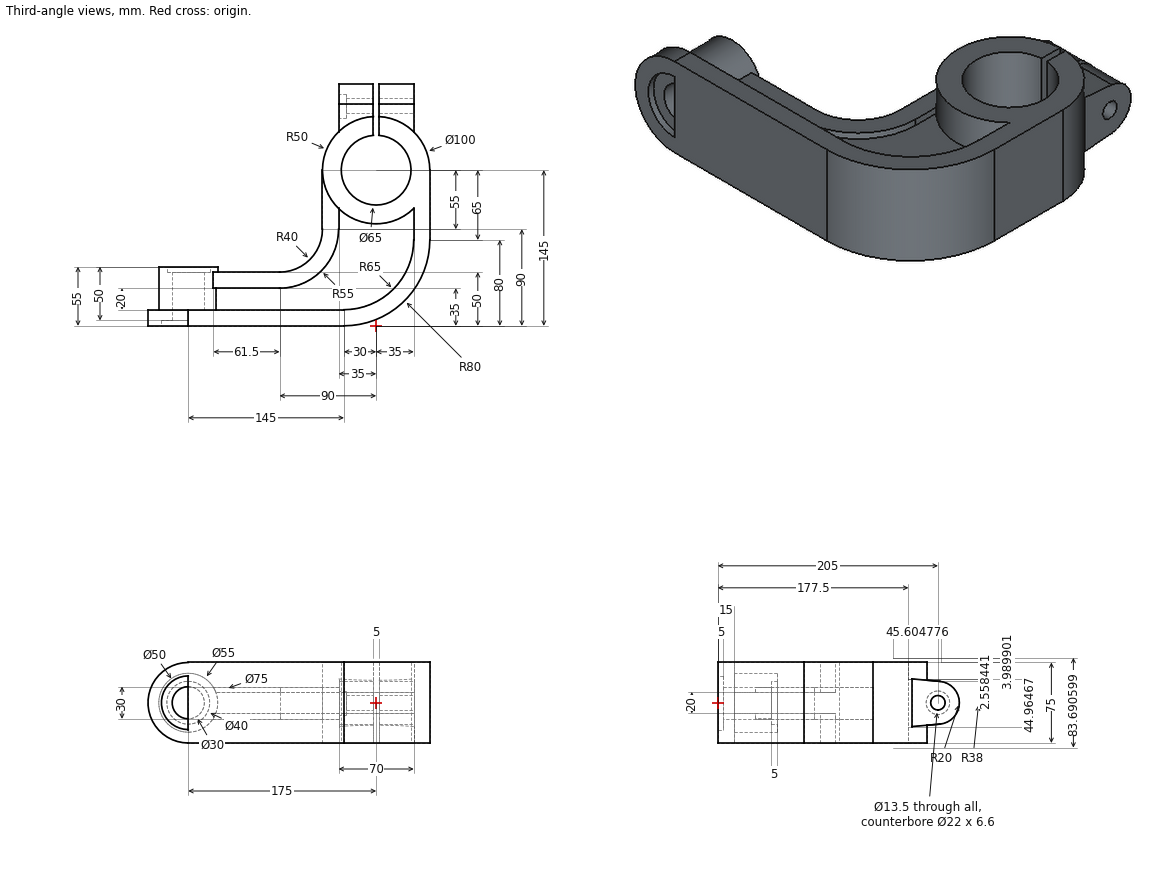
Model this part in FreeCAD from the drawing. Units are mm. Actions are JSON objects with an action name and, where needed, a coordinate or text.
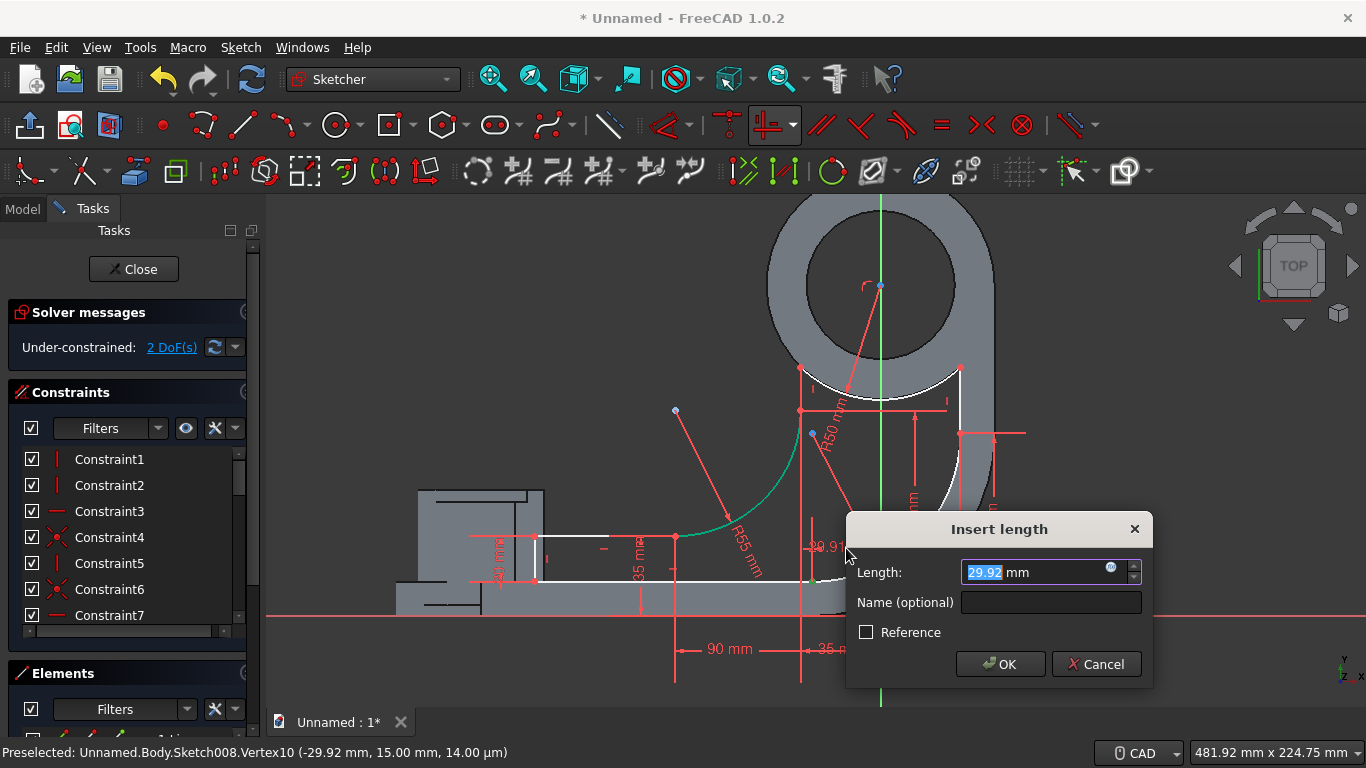
{"action": "type", "text": "30"}
{"action": "key", "text": "Return"}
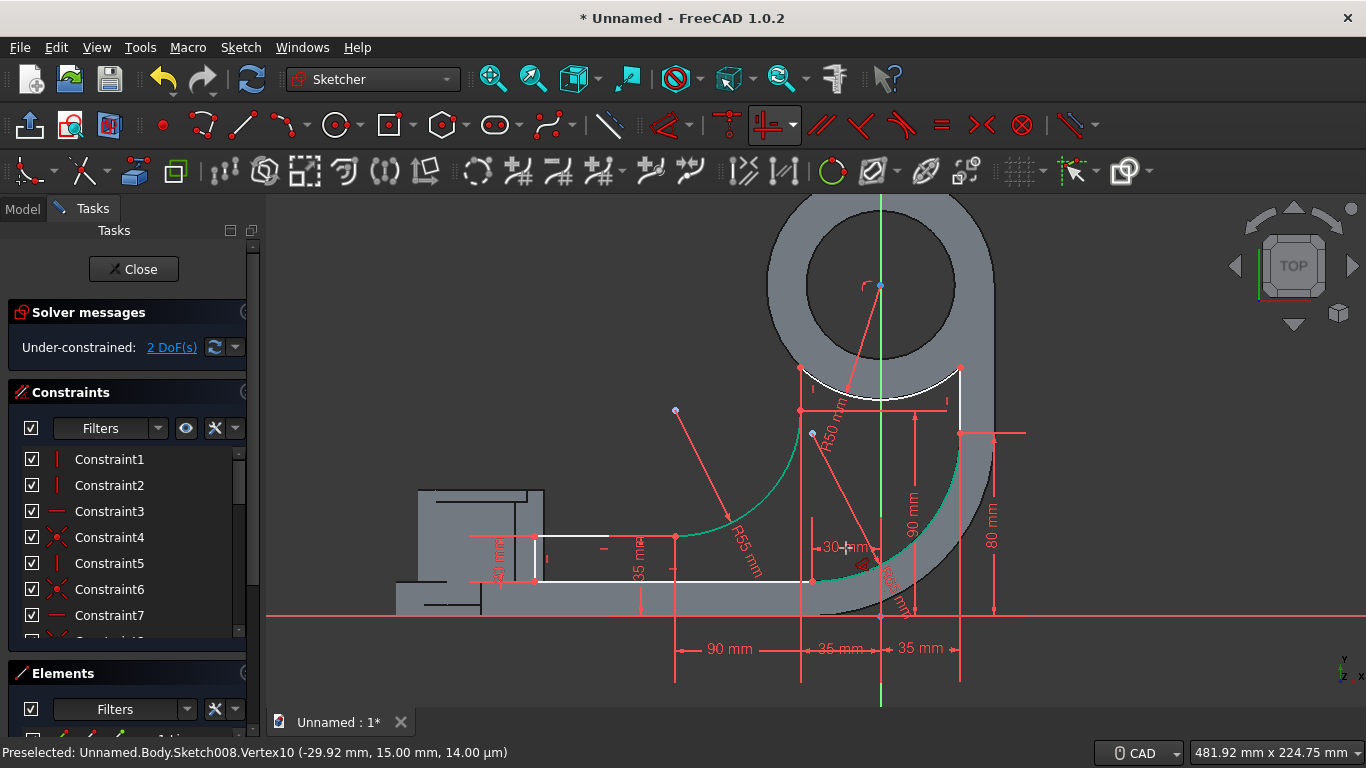
{"action": "left_click", "coordinate": [633, 536]}
{"action": "left_click", "coordinate": [605, 502]}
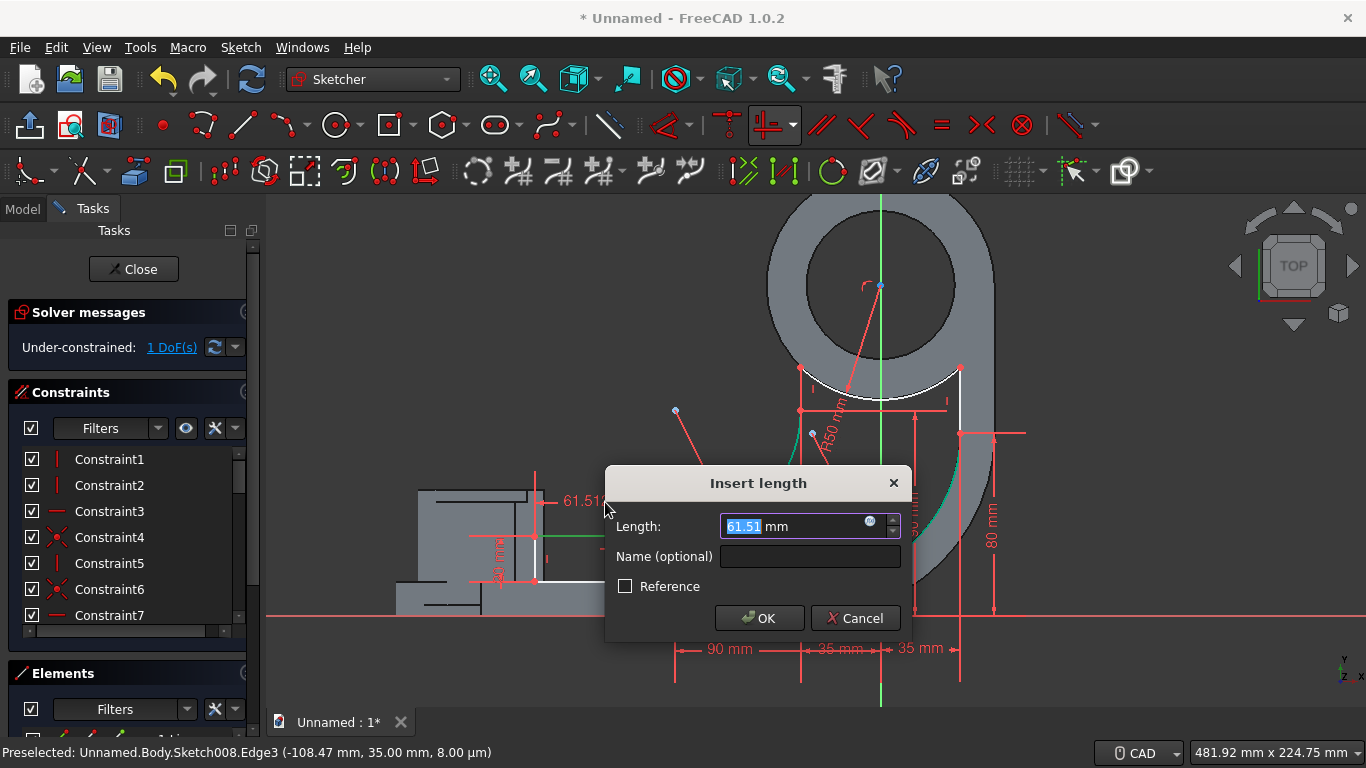
{"action": "type", "text": "61.5"}
{"action": "key", "text": "Return"}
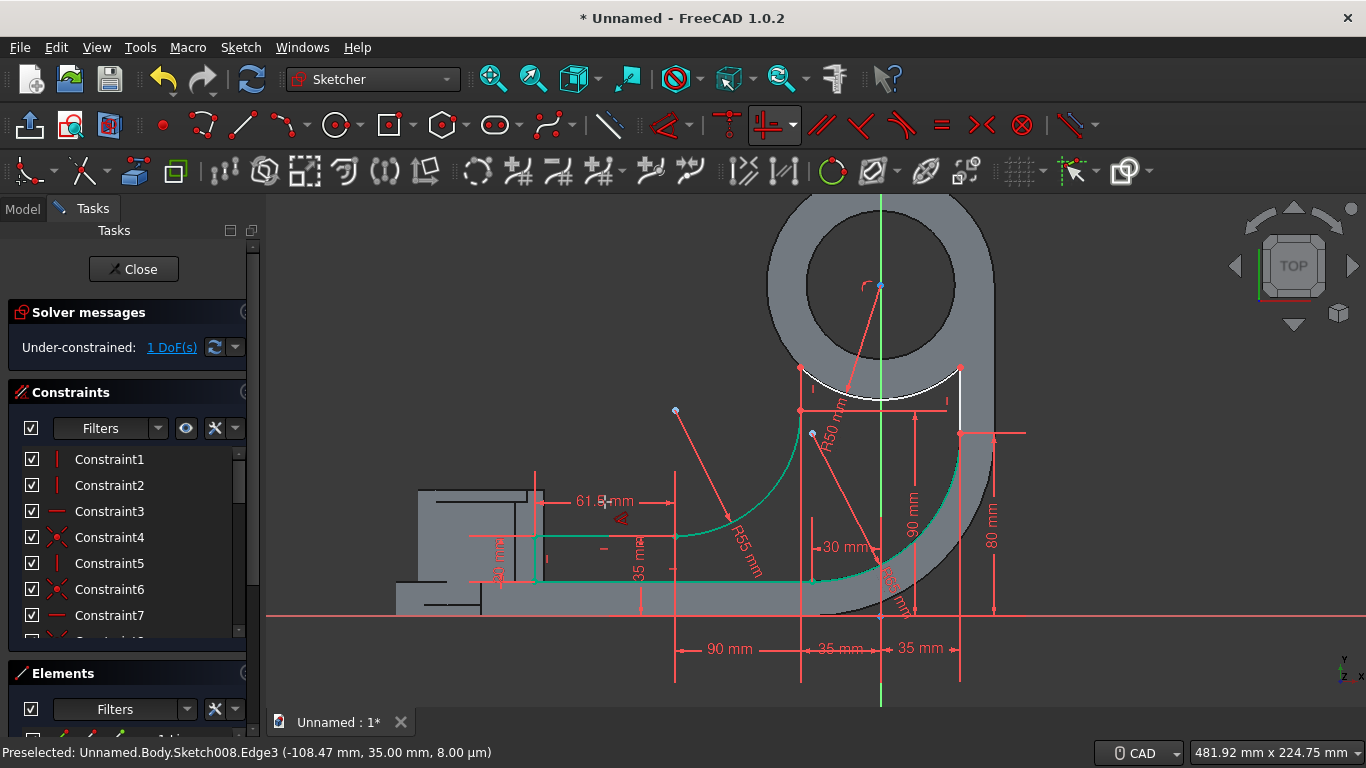
{"action": "left_click", "coordinate": [881, 286]}
{"action": "left_click", "coordinate": [915, 451]}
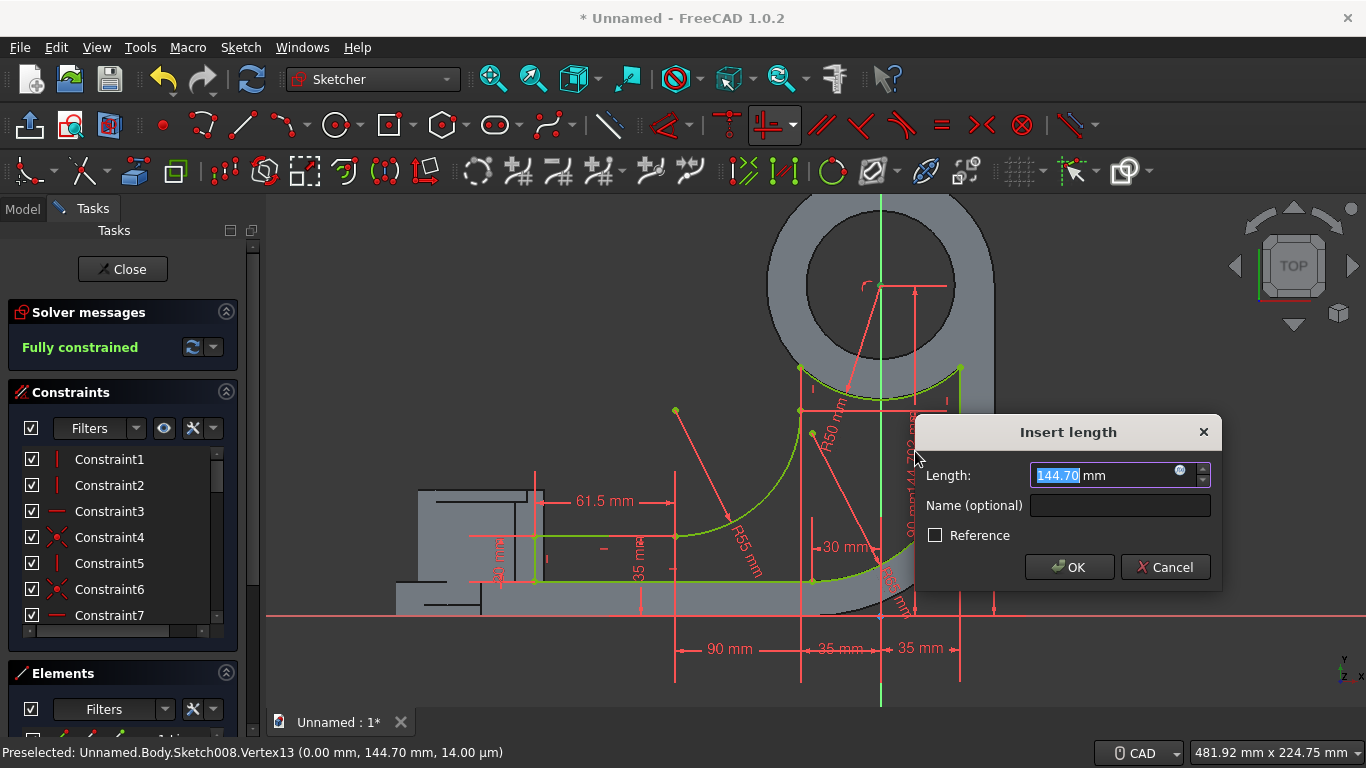
{"action": "type", "text": "145"}
{"action": "key", "text": "Return"}
{"action": "key", "text": "Escape"}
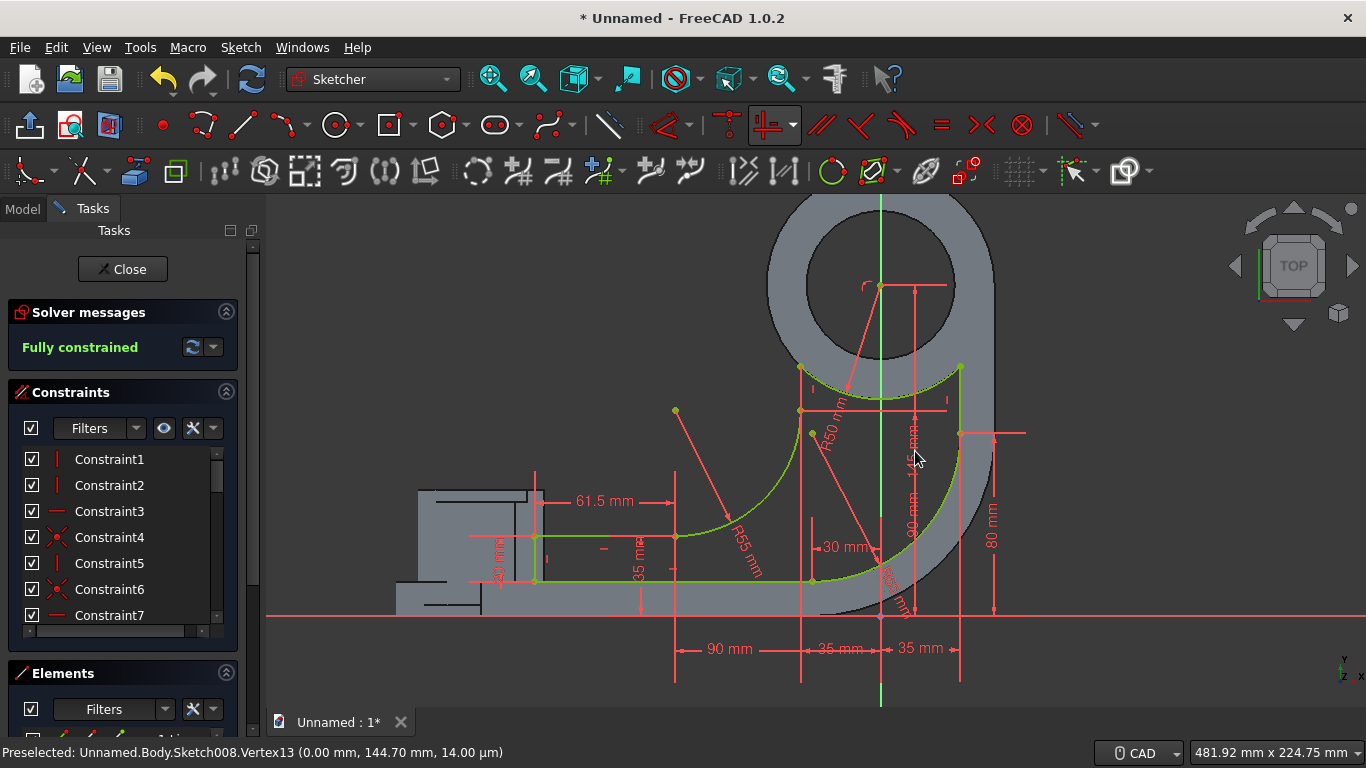
{"action": "left_click", "coordinate": [123, 269]}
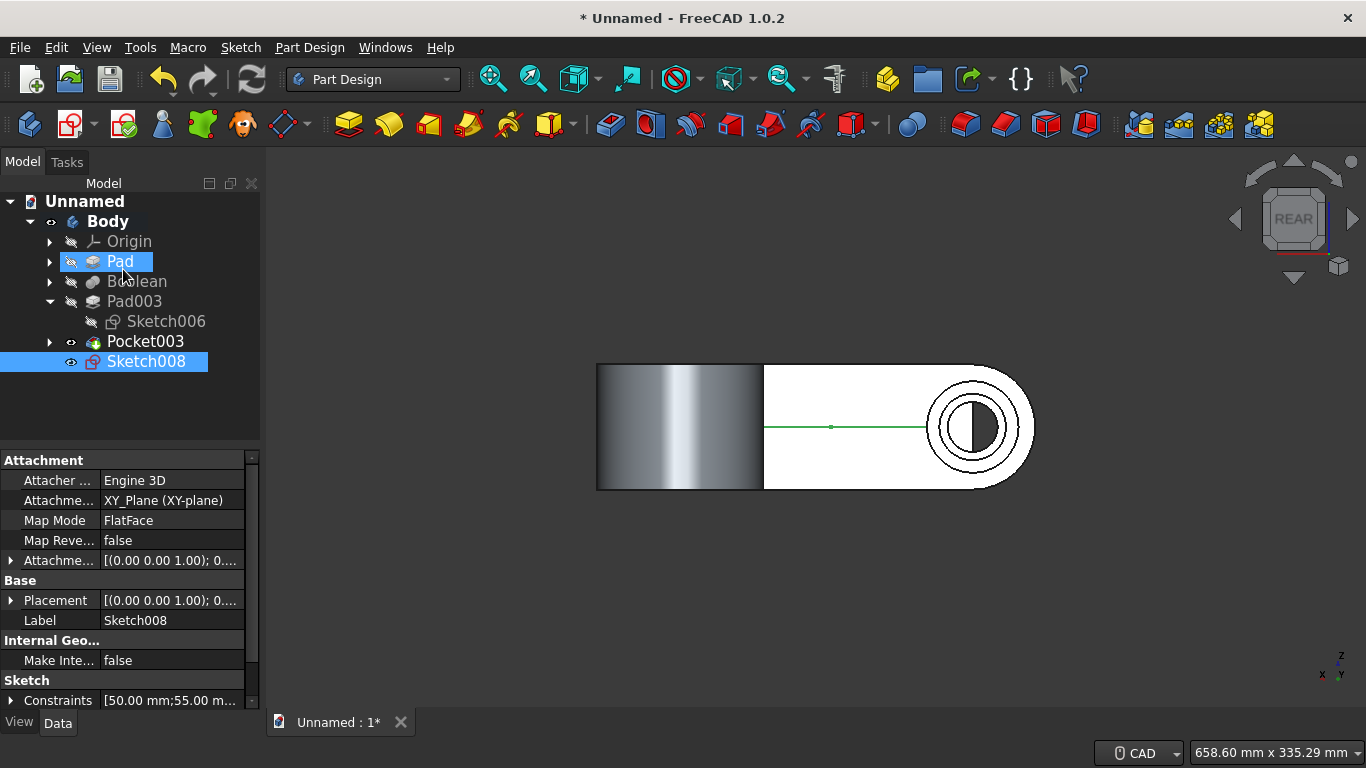
{"action": "left_click", "coordinate": [350, 124]}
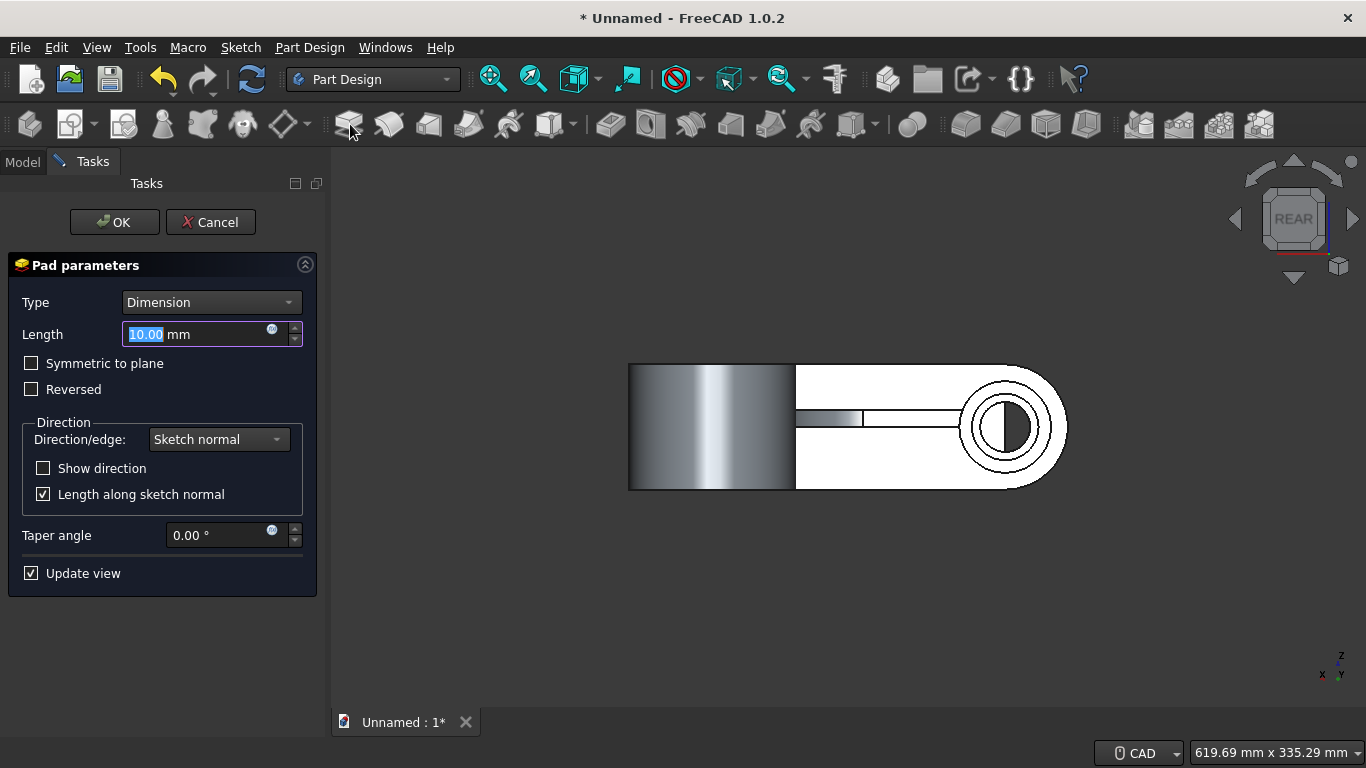
{"action": "type", "text": "20"}
{"action": "key", "text": "Tab"}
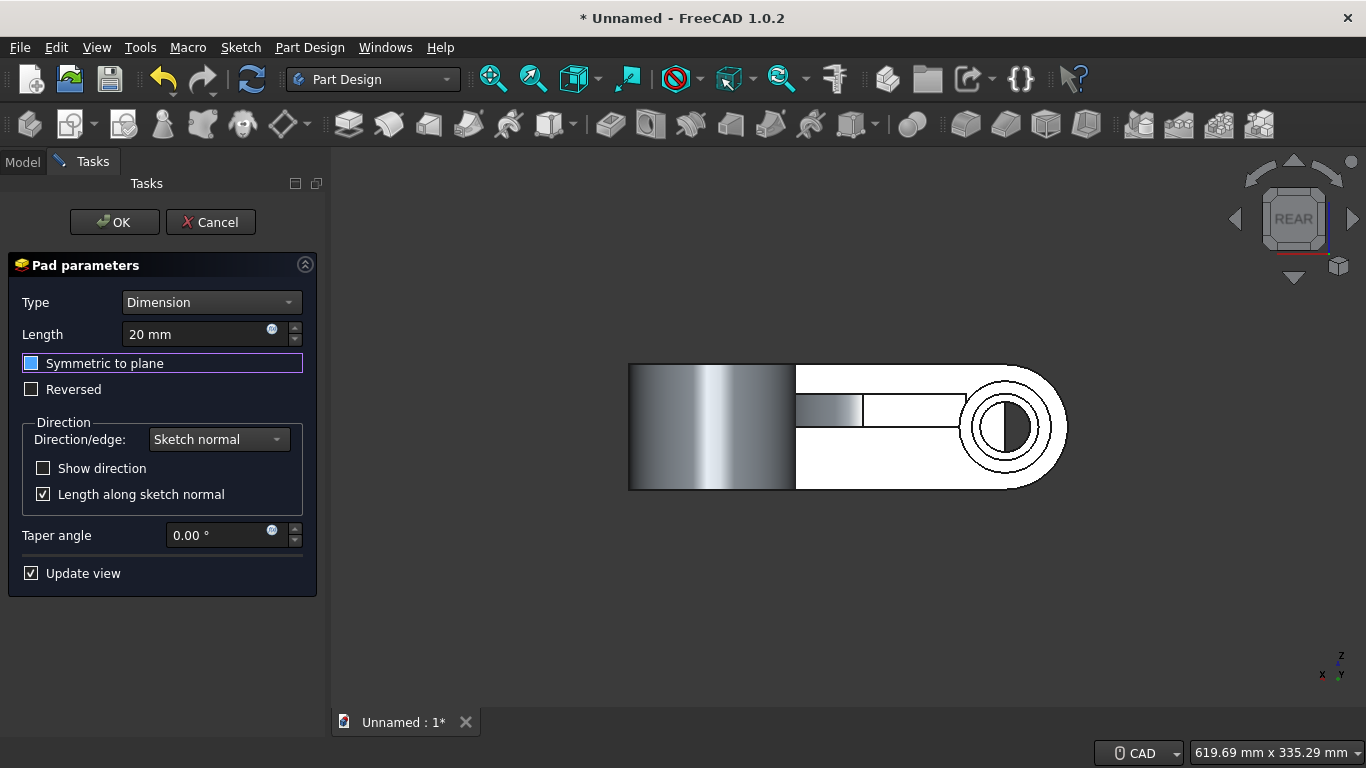
{"action": "left_click", "coordinate": [30, 363]}